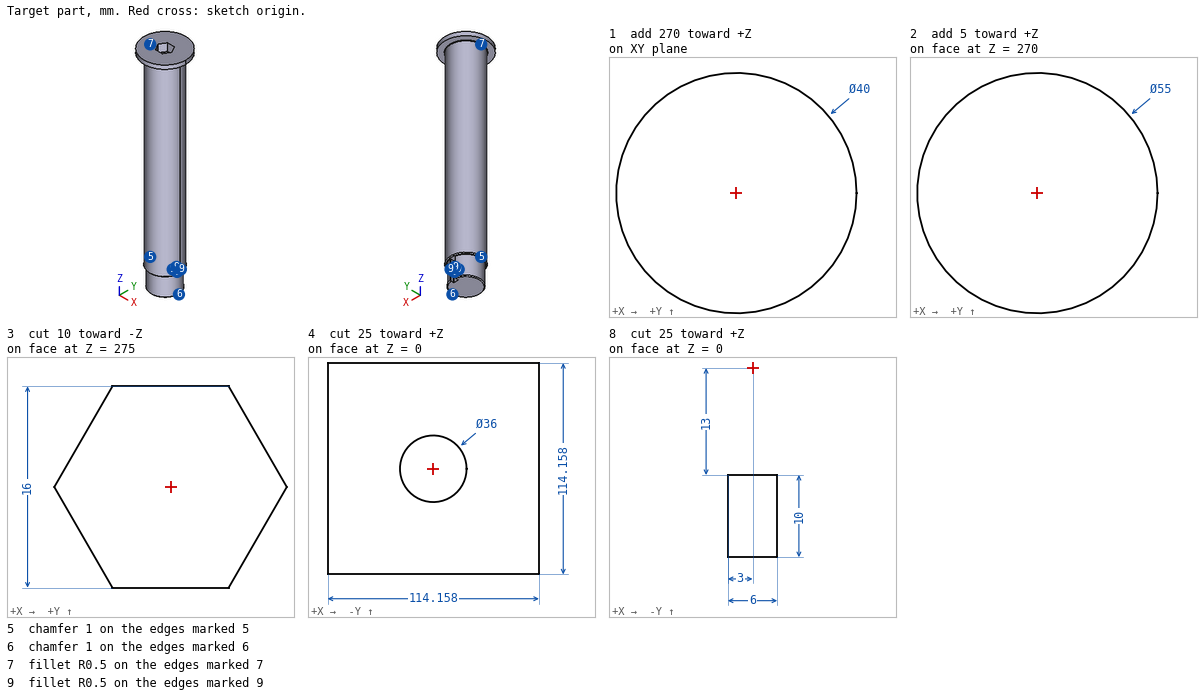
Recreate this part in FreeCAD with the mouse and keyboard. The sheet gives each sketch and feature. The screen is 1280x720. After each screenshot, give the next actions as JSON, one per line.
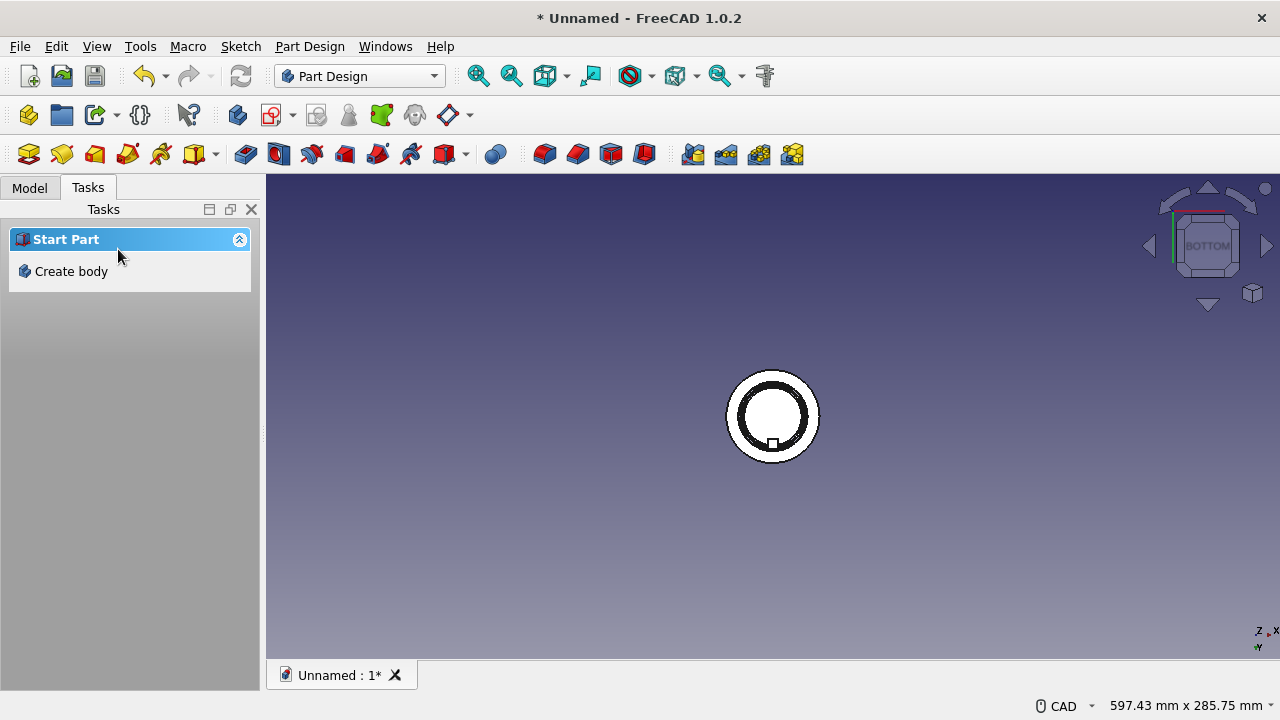
{"action": "left_click", "coordinate": [479, 76]}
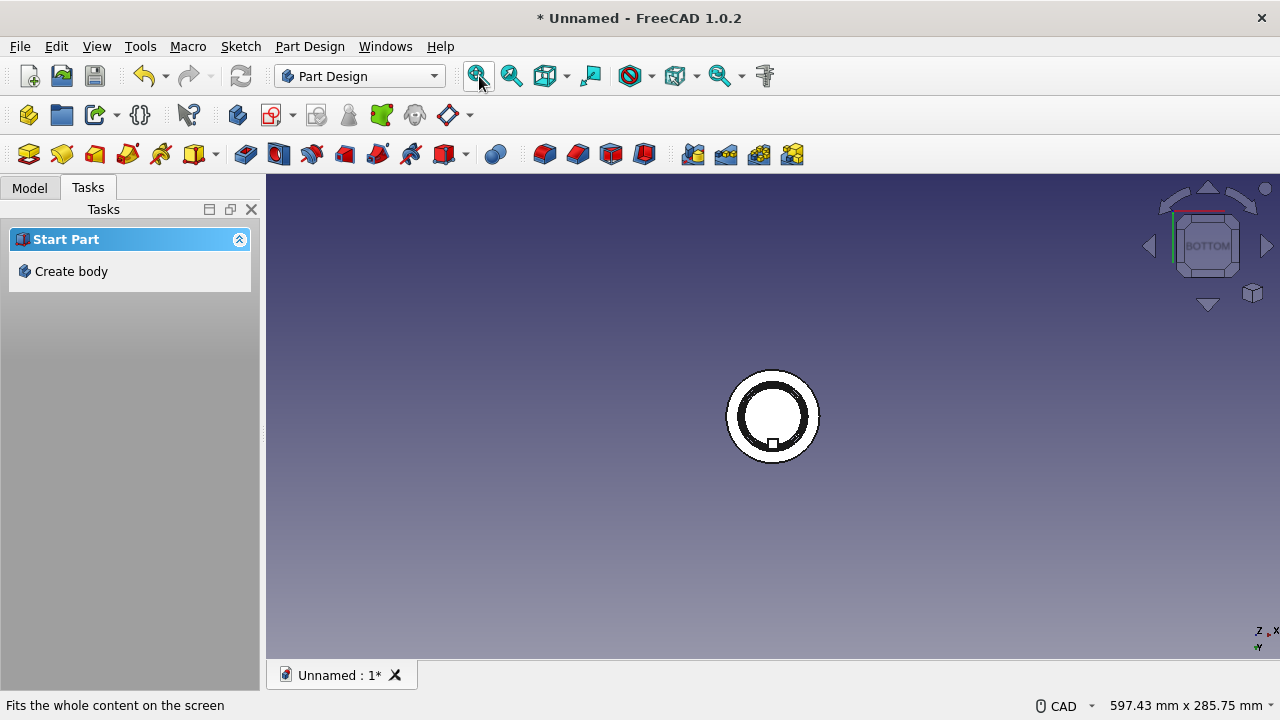
{"action": "key", "text": "0"}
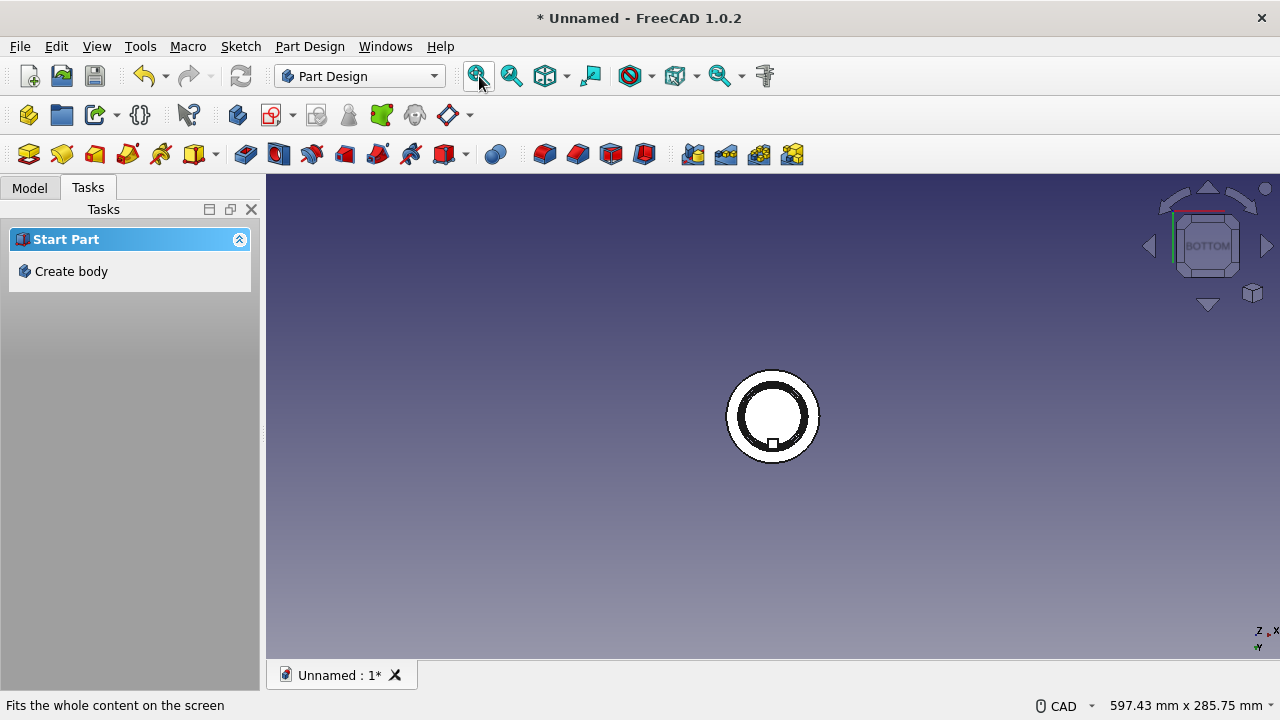
{"action": "key", "text": "2"}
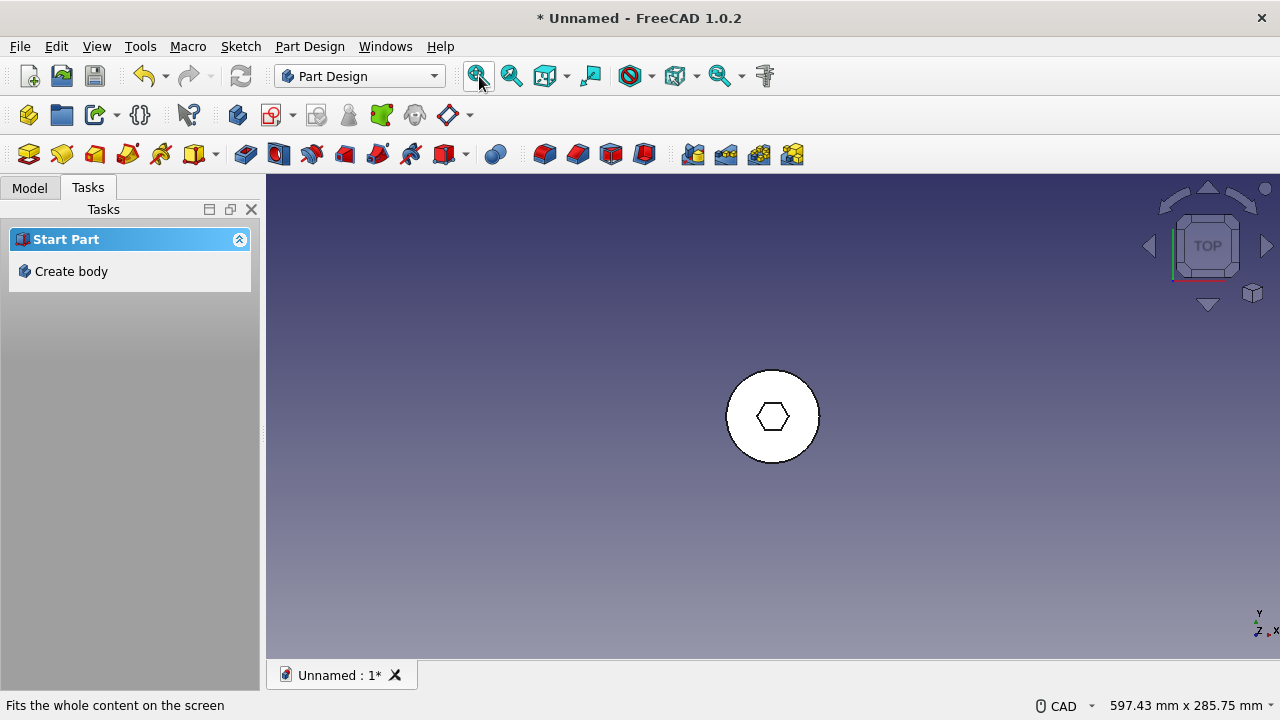
{"action": "left_click", "coordinate": [479, 76]}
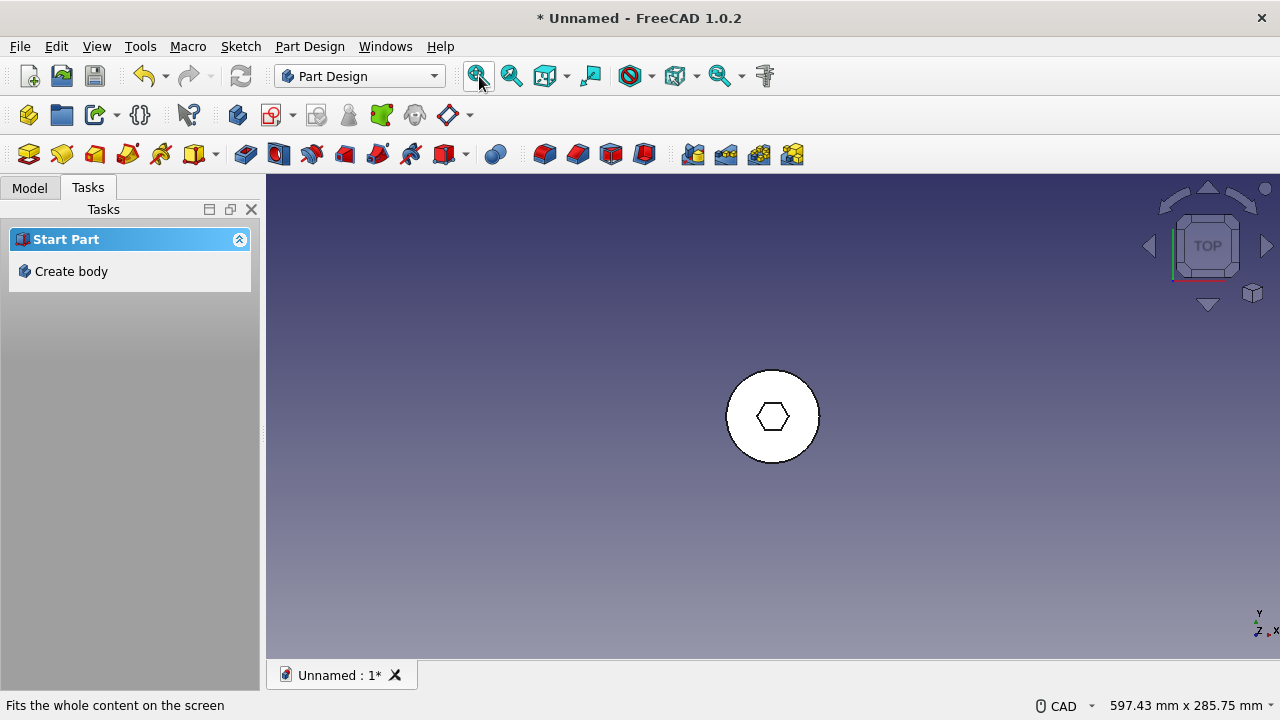
{"action": "key", "text": "1"}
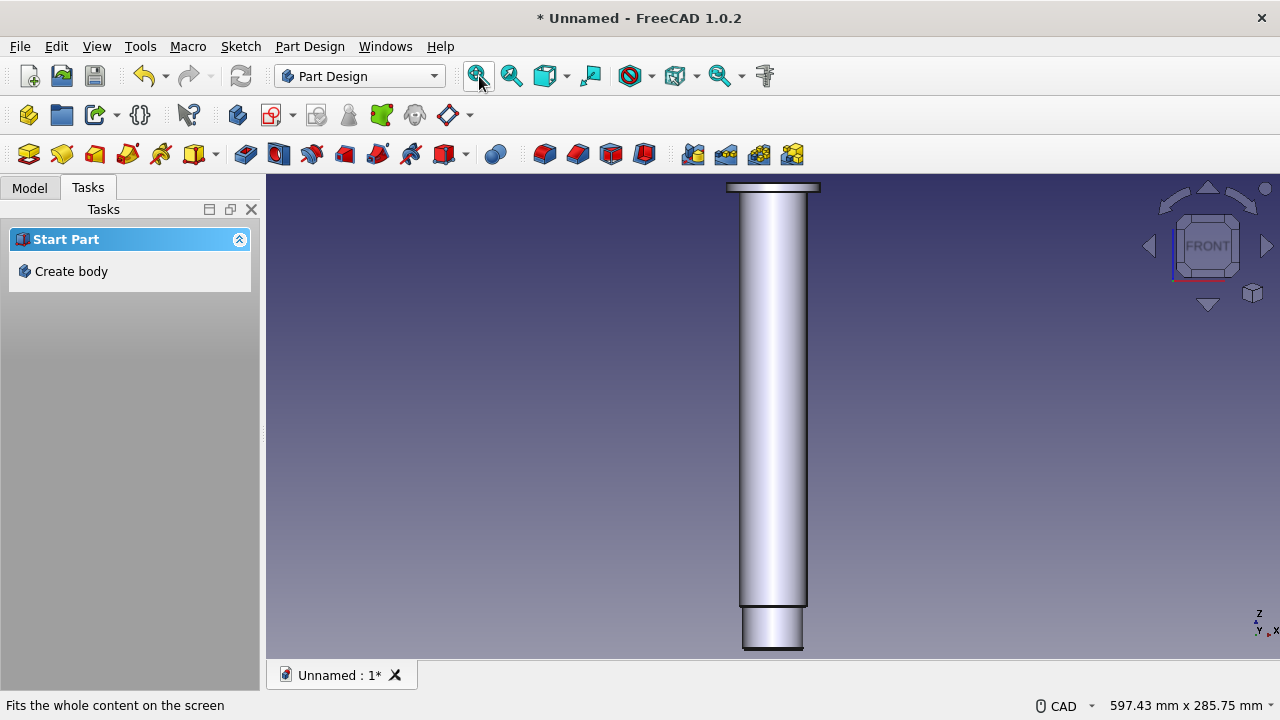
{"action": "key", "text": "3"}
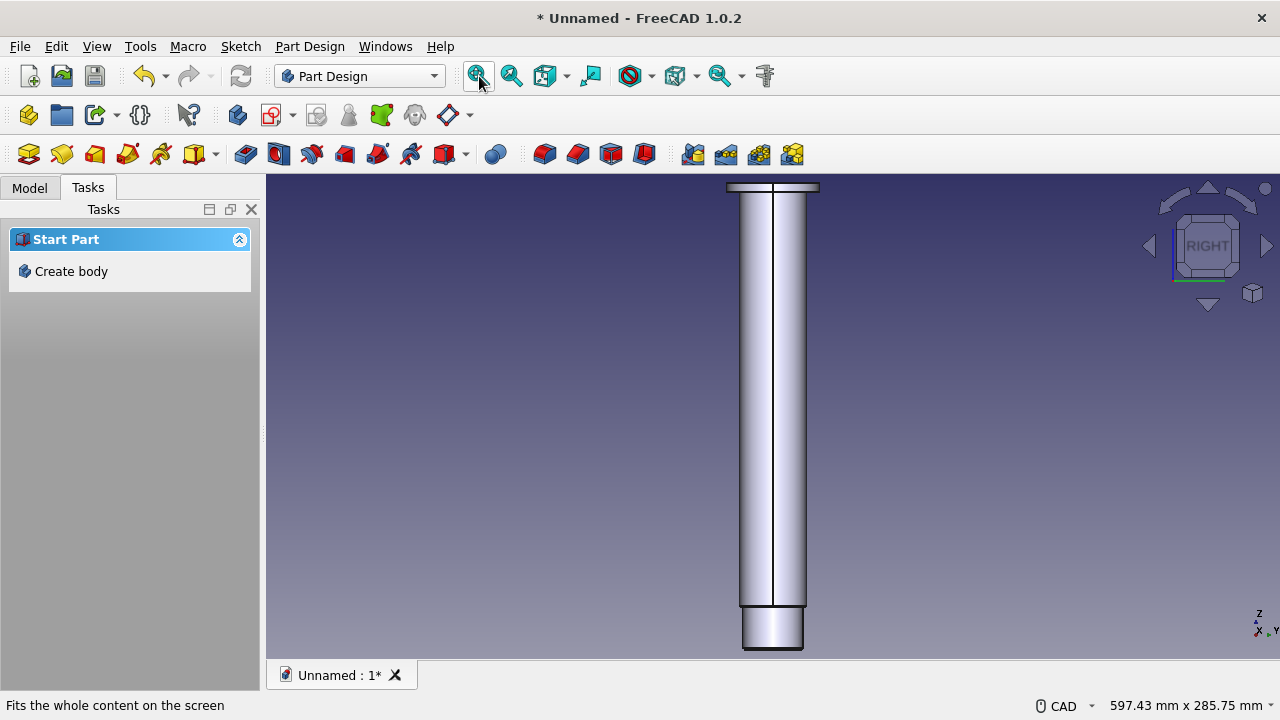
{"action": "key", "text": "5"}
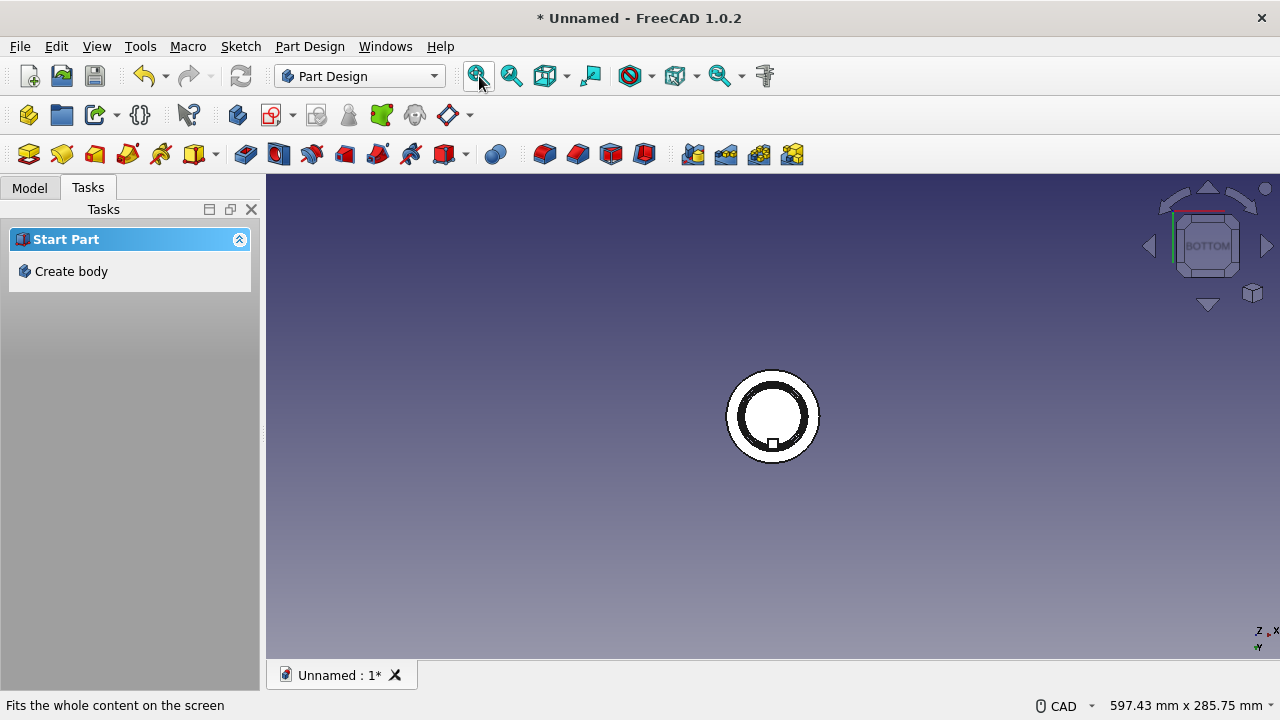
{"action": "left_click", "coordinate": [479, 76]}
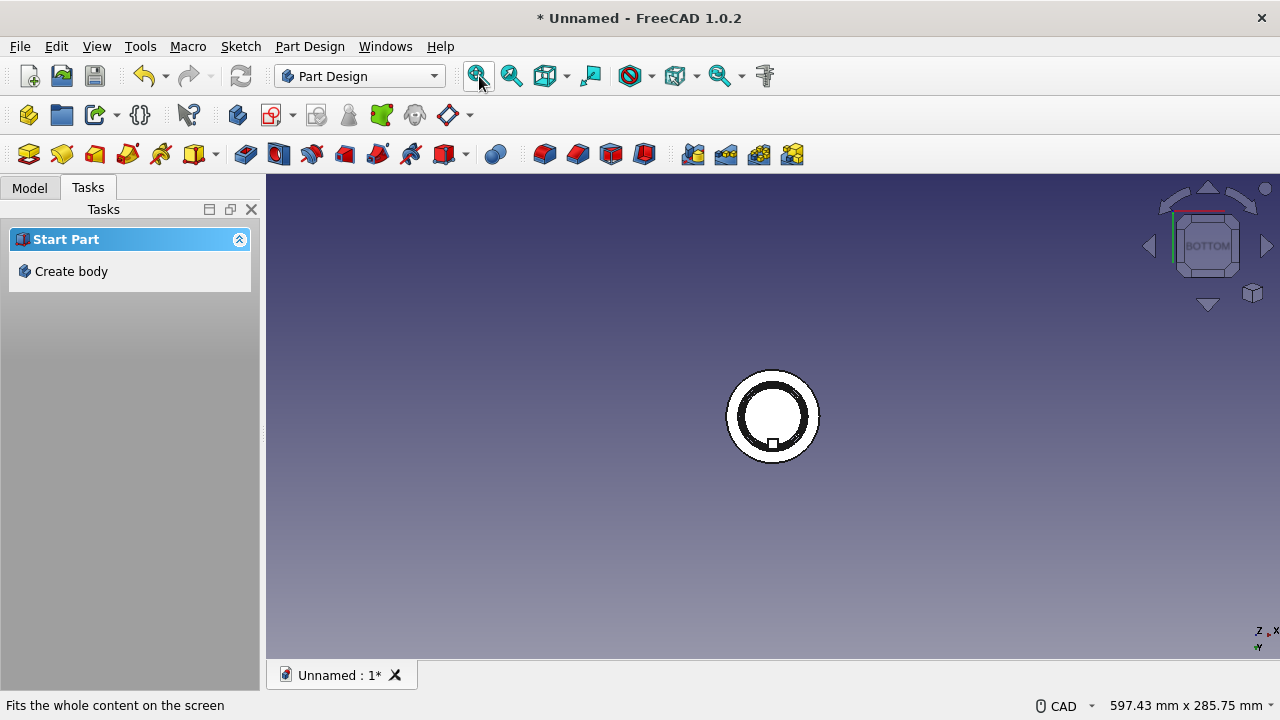
{"action": "key", "text": "4"}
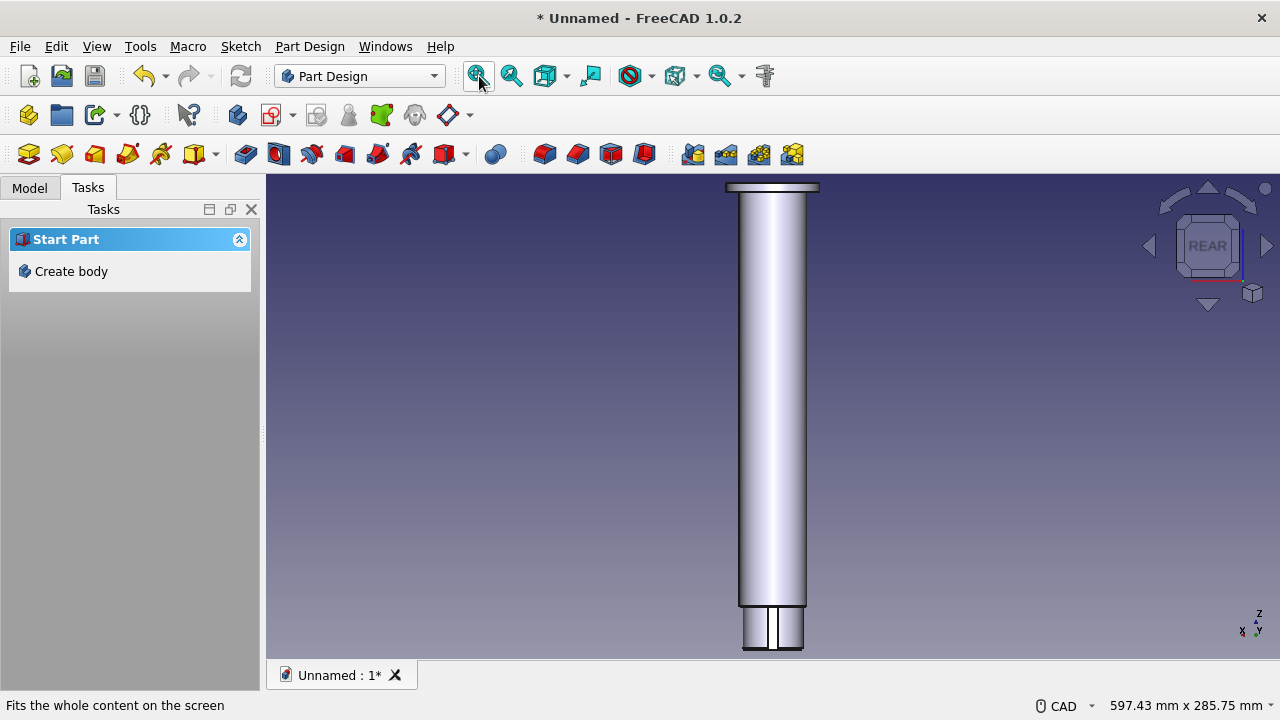
{"action": "left_click", "coordinate": [778, 627]}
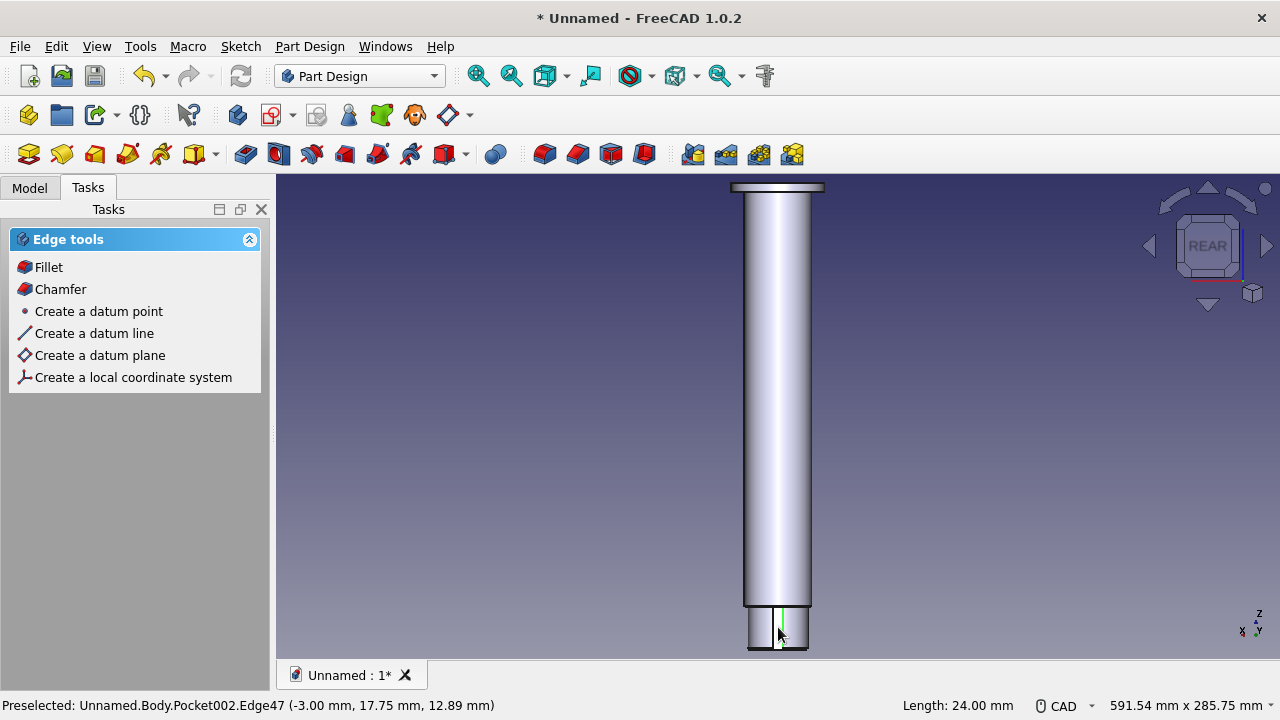
{"action": "left_click", "coordinate": [773, 627], "text": "ctrl"}